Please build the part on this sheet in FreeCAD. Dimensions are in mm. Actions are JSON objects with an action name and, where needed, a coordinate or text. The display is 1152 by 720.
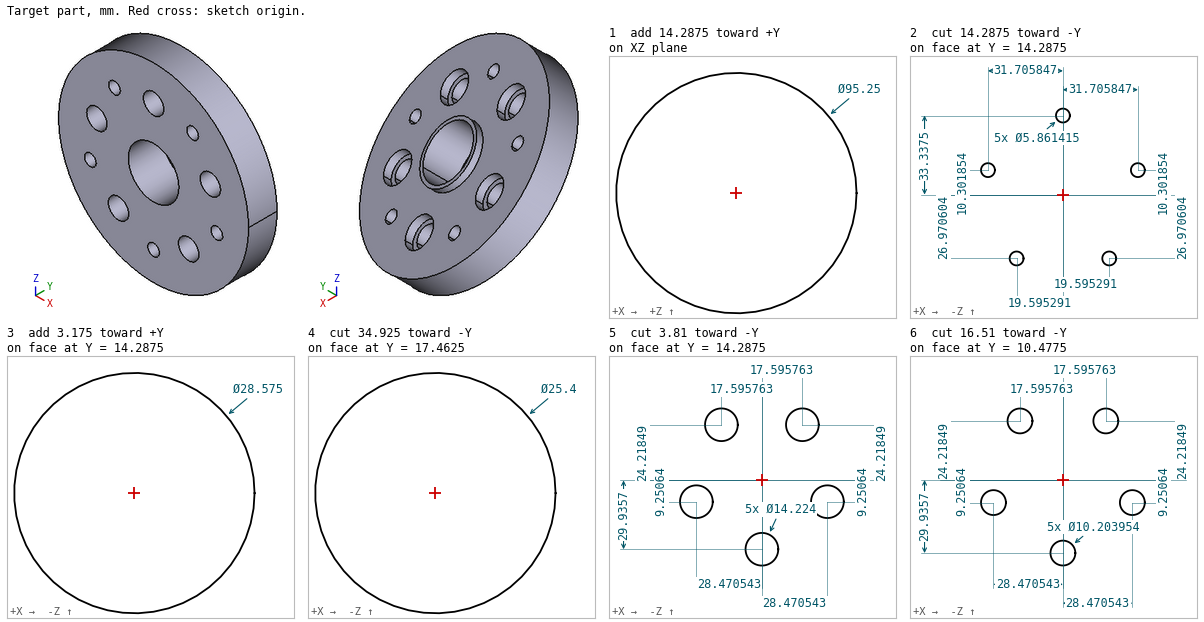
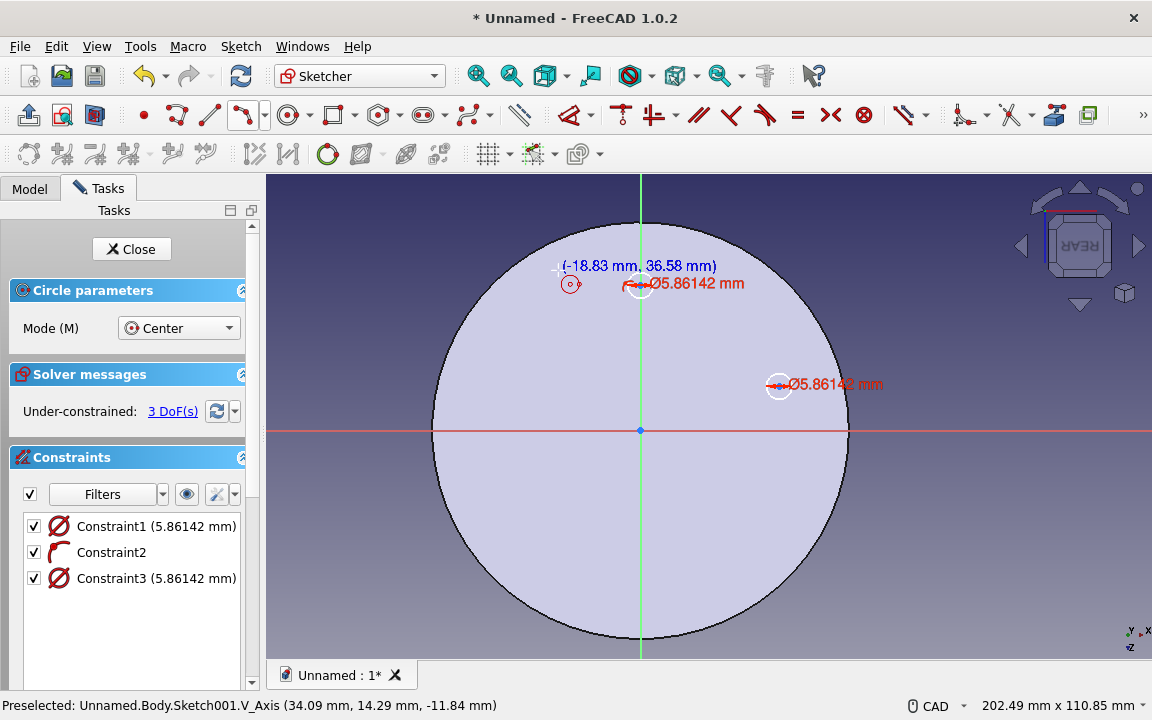
{"action": "scroll", "coordinate": [726, 549], "scroll_direction": "up", "scroll_amount": 3}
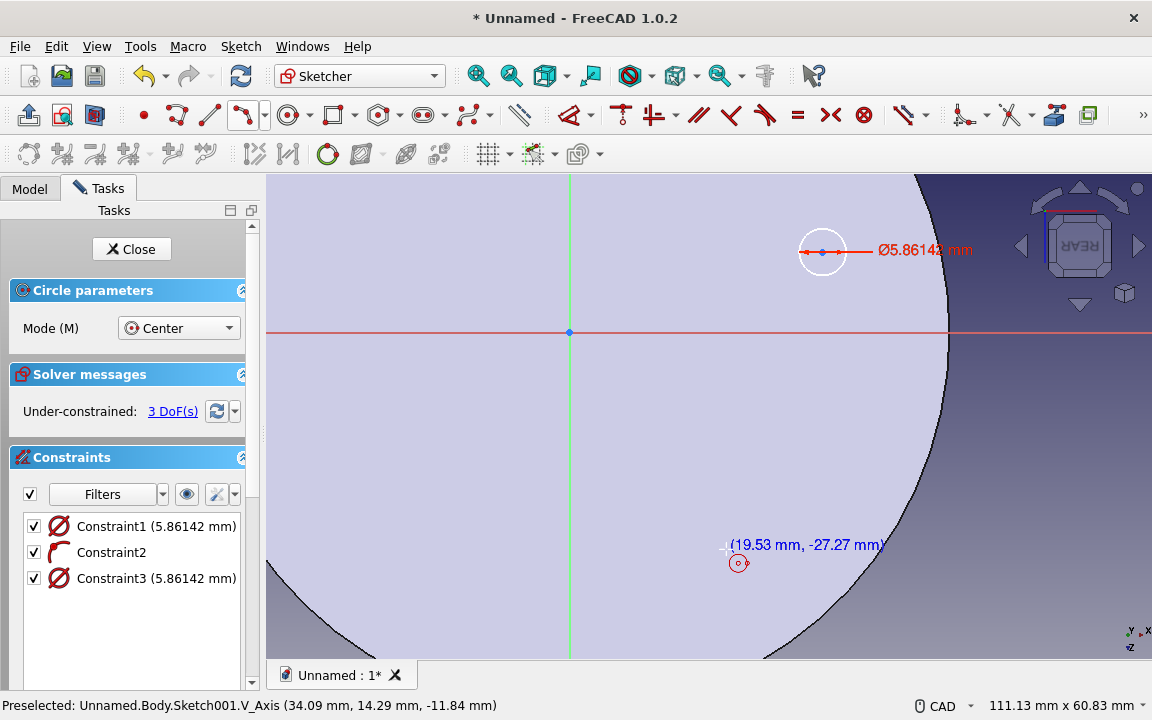
{"action": "left_click", "coordinate": [726, 548]}
{"action": "mouse_move", "coordinate": [743, 531]}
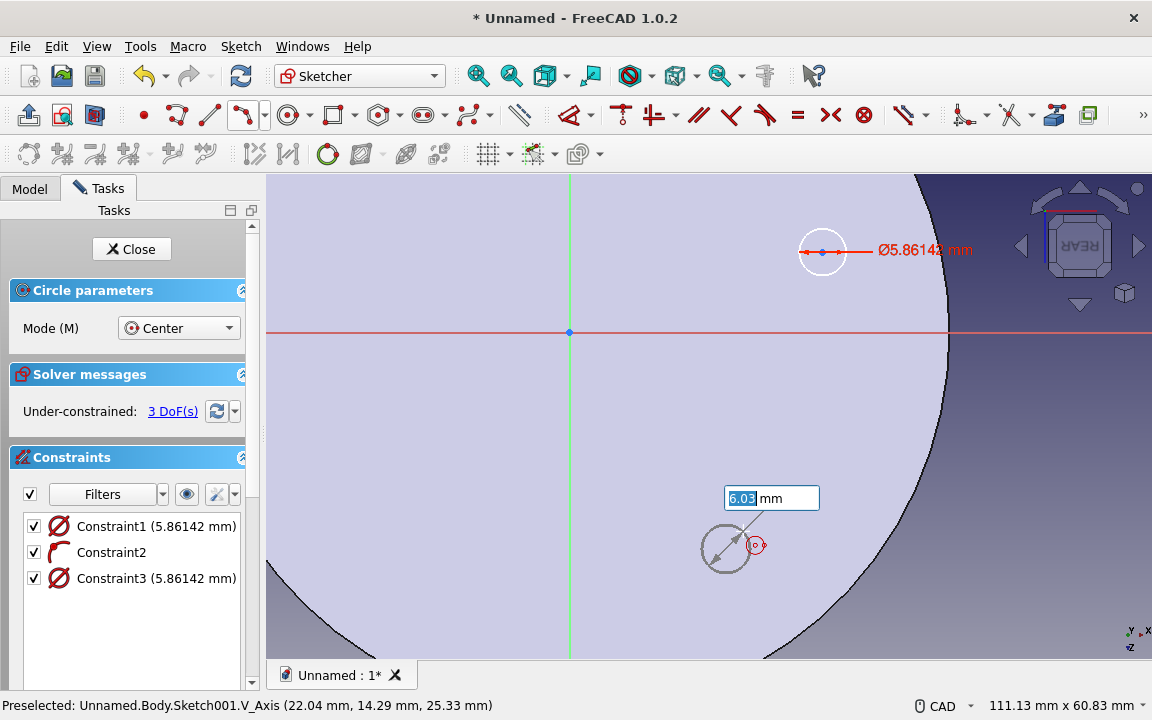
{"action": "type", "text": "5.861415"}
{"action": "key", "text": "Return"}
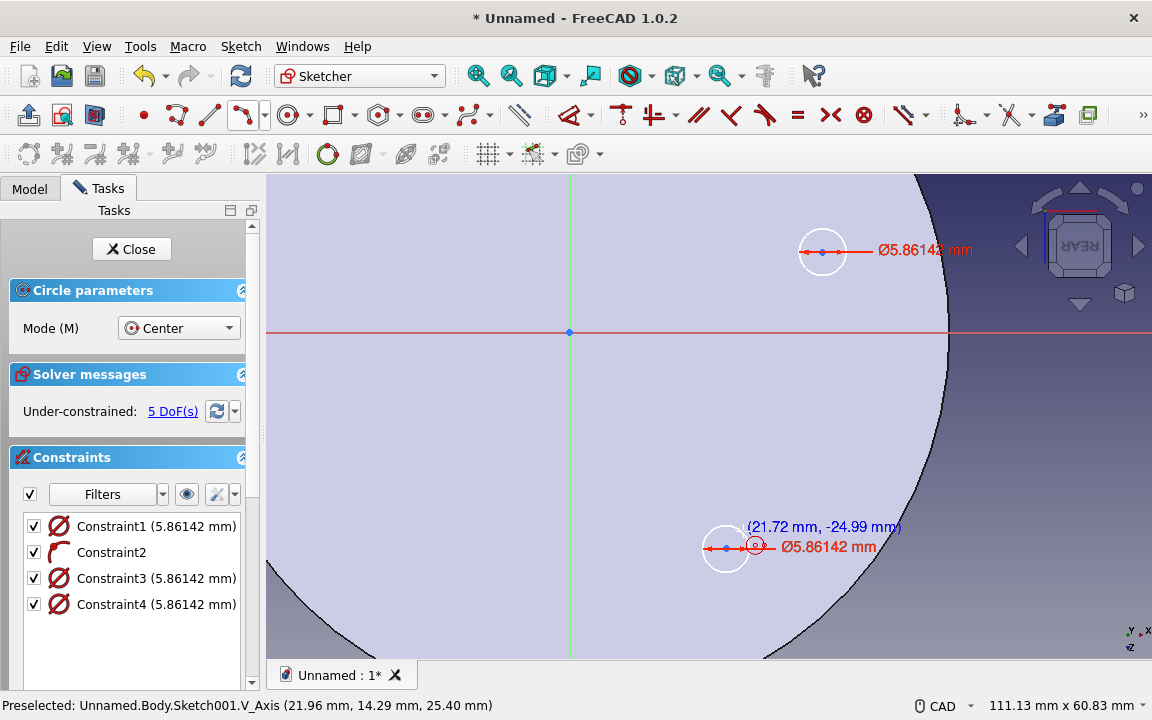
{"action": "left_click", "coordinate": [414, 548]}
{"action": "mouse_move", "coordinate": [430, 531]}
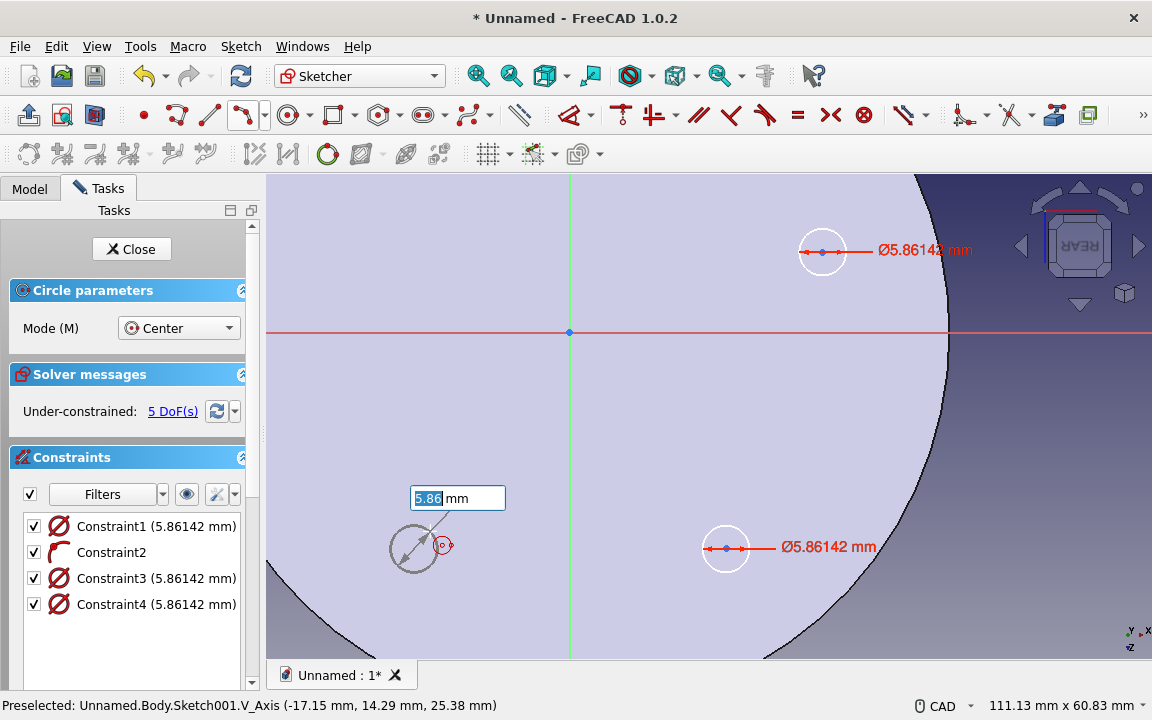
{"action": "type", "text": "5.861415"}
{"action": "key", "text": "Return"}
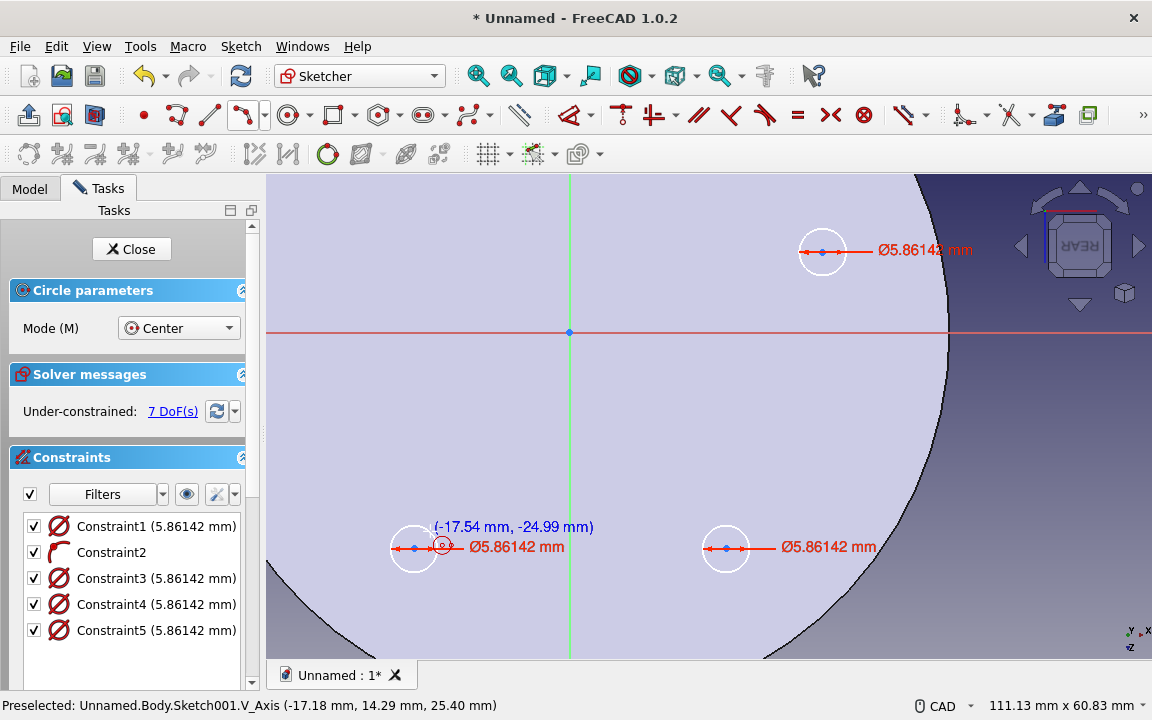
{"action": "left_click", "coordinate": [317, 251]}
{"action": "mouse_move", "coordinate": [334, 234]}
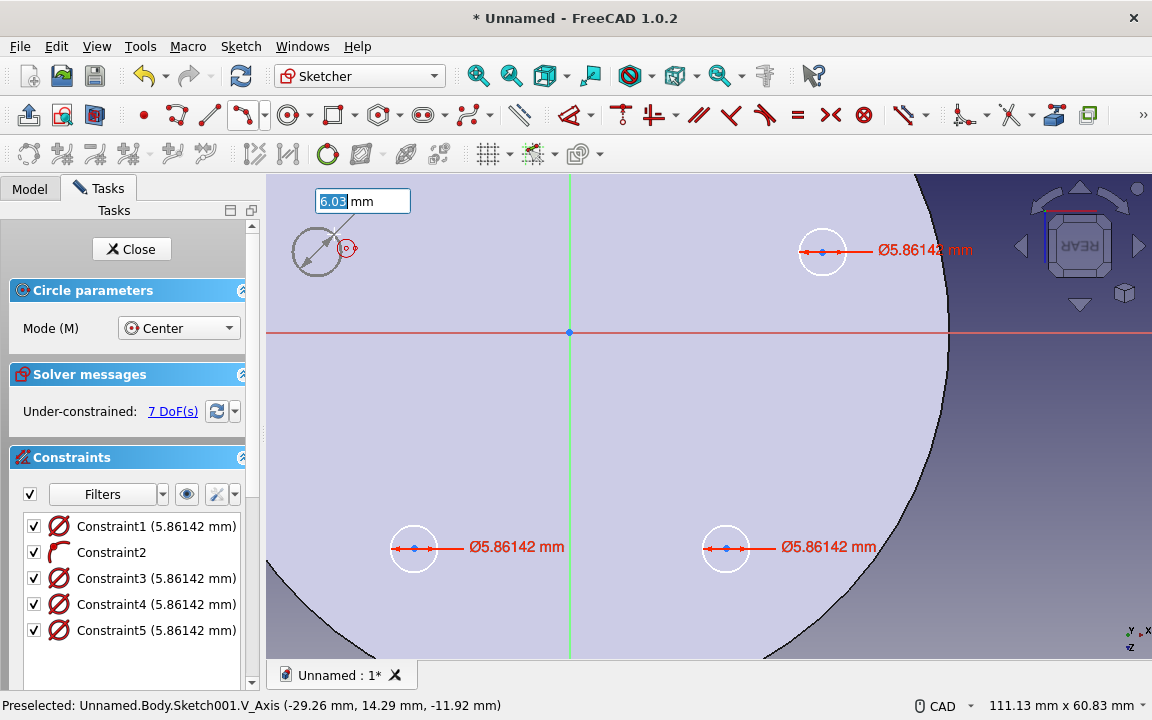
{"action": "type", "text": "5.861415"}
{"action": "key", "text": "Return"}
{"action": "key", "text": "Escape"}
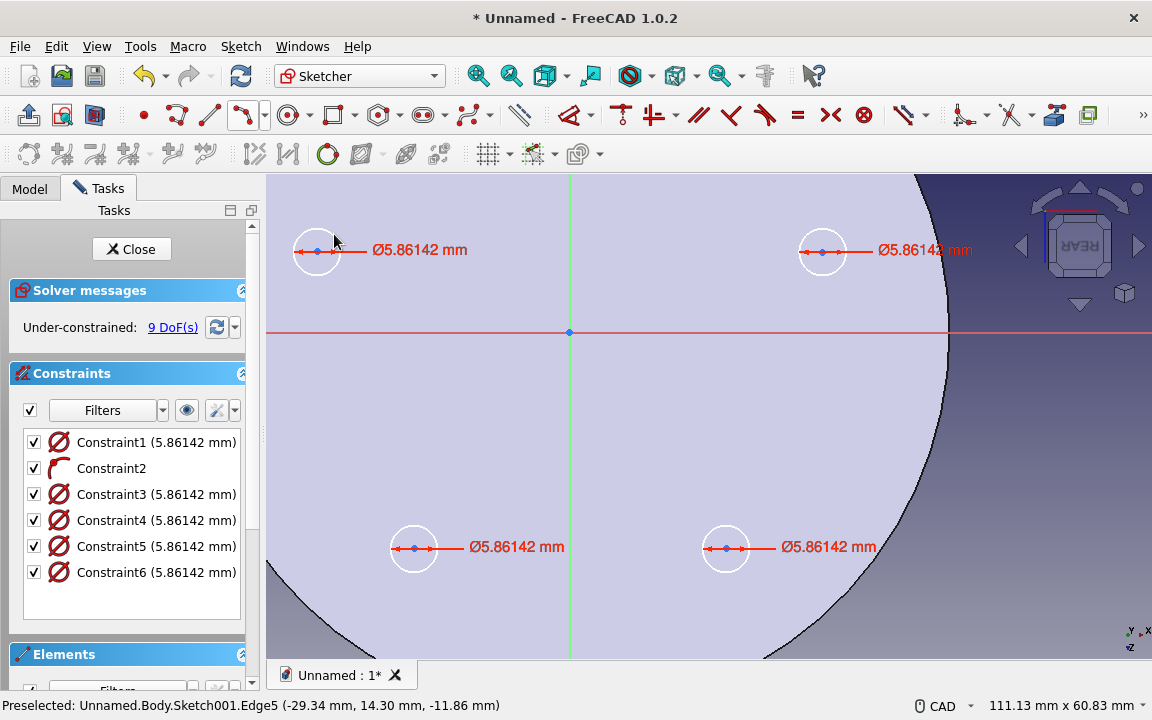
{"action": "left_click", "coordinate": [568, 116]}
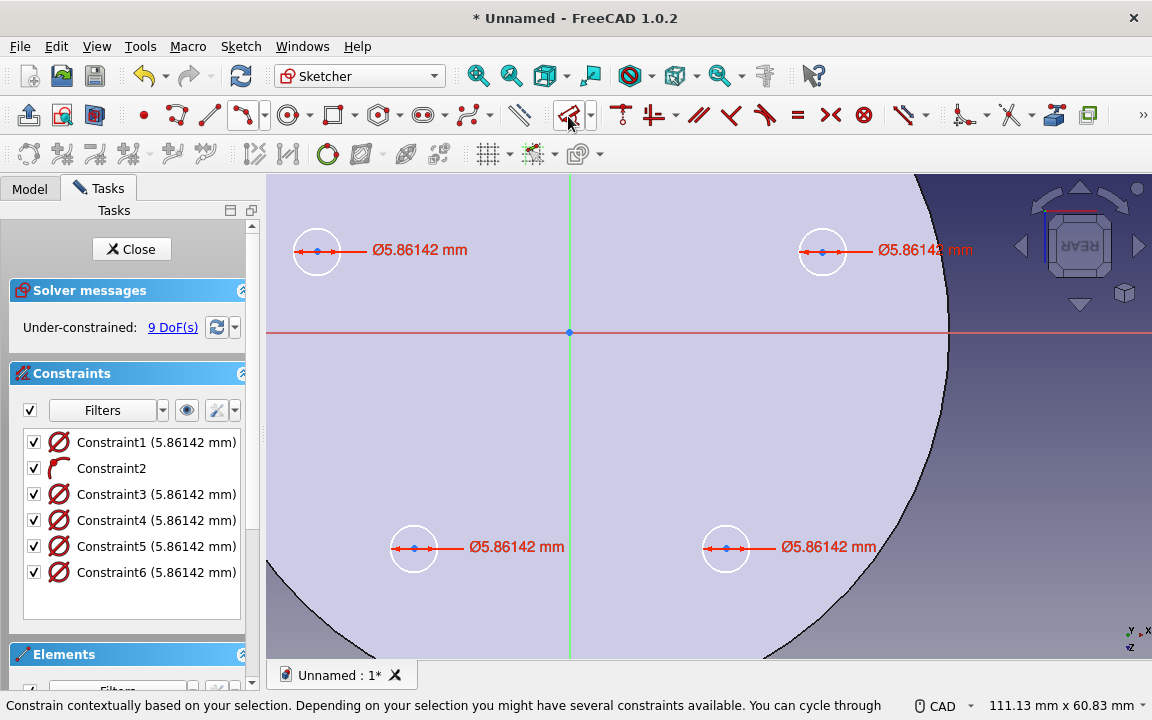
{"action": "scroll", "coordinate": [726, 549], "scroll_direction": "down", "scroll_amount": 3}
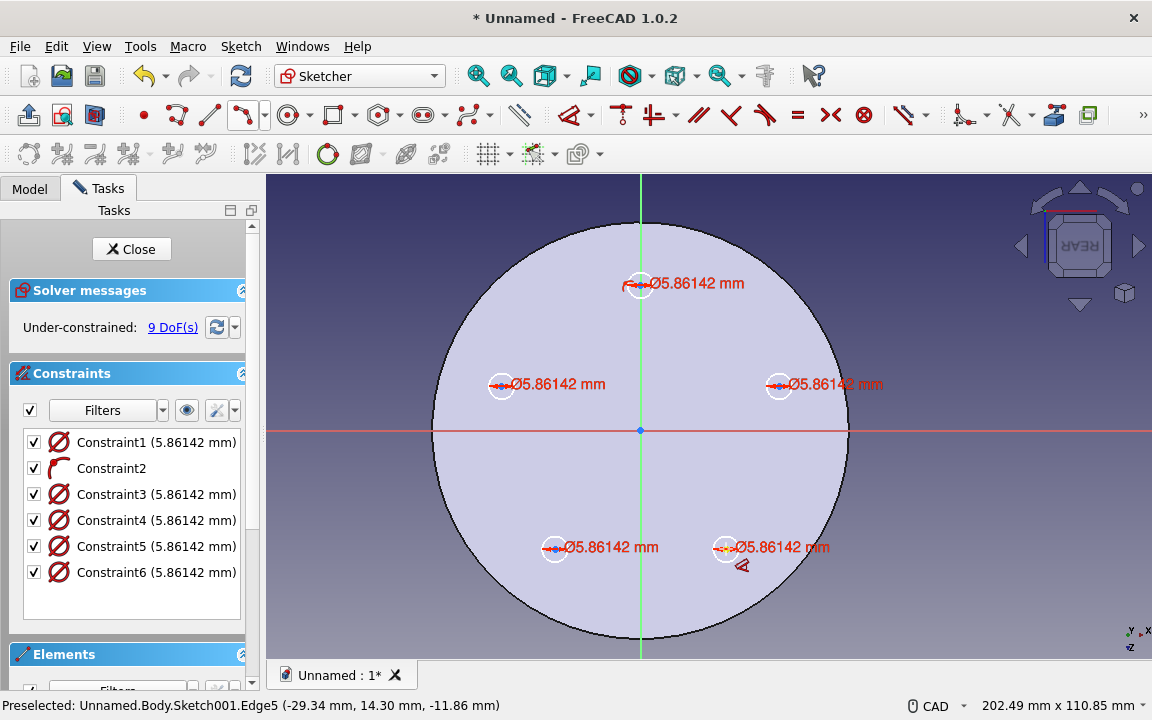
{"action": "left_click", "coordinate": [641, 285]}
{"action": "left_click", "coordinate": [675, 358]}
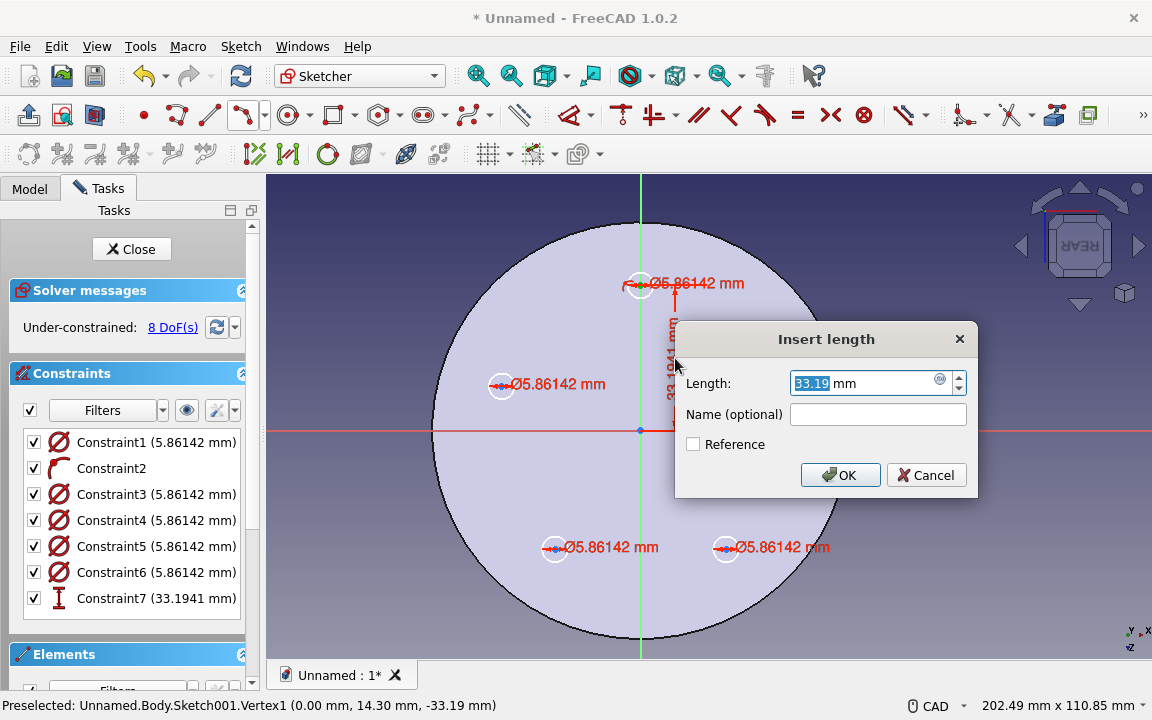
{"action": "type", "text": "33.3375"}
{"action": "key", "text": "Return"}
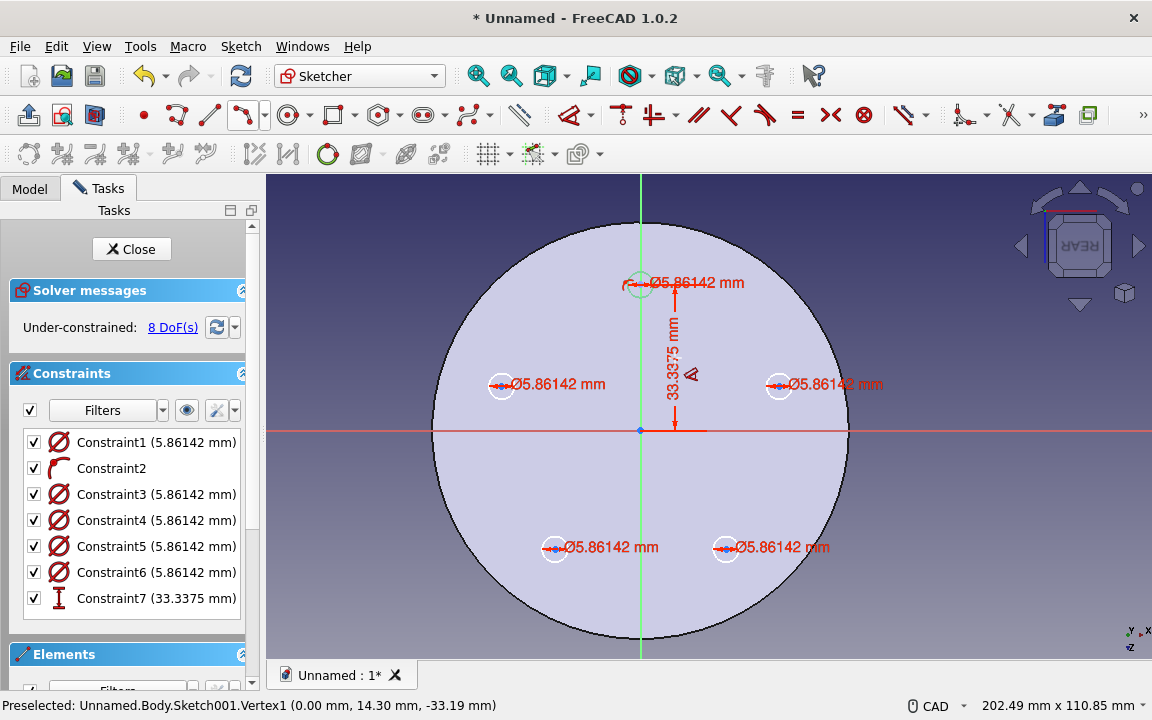
{"action": "left_click", "coordinate": [779, 386]}
{"action": "left_click", "coordinate": [759, 352]}